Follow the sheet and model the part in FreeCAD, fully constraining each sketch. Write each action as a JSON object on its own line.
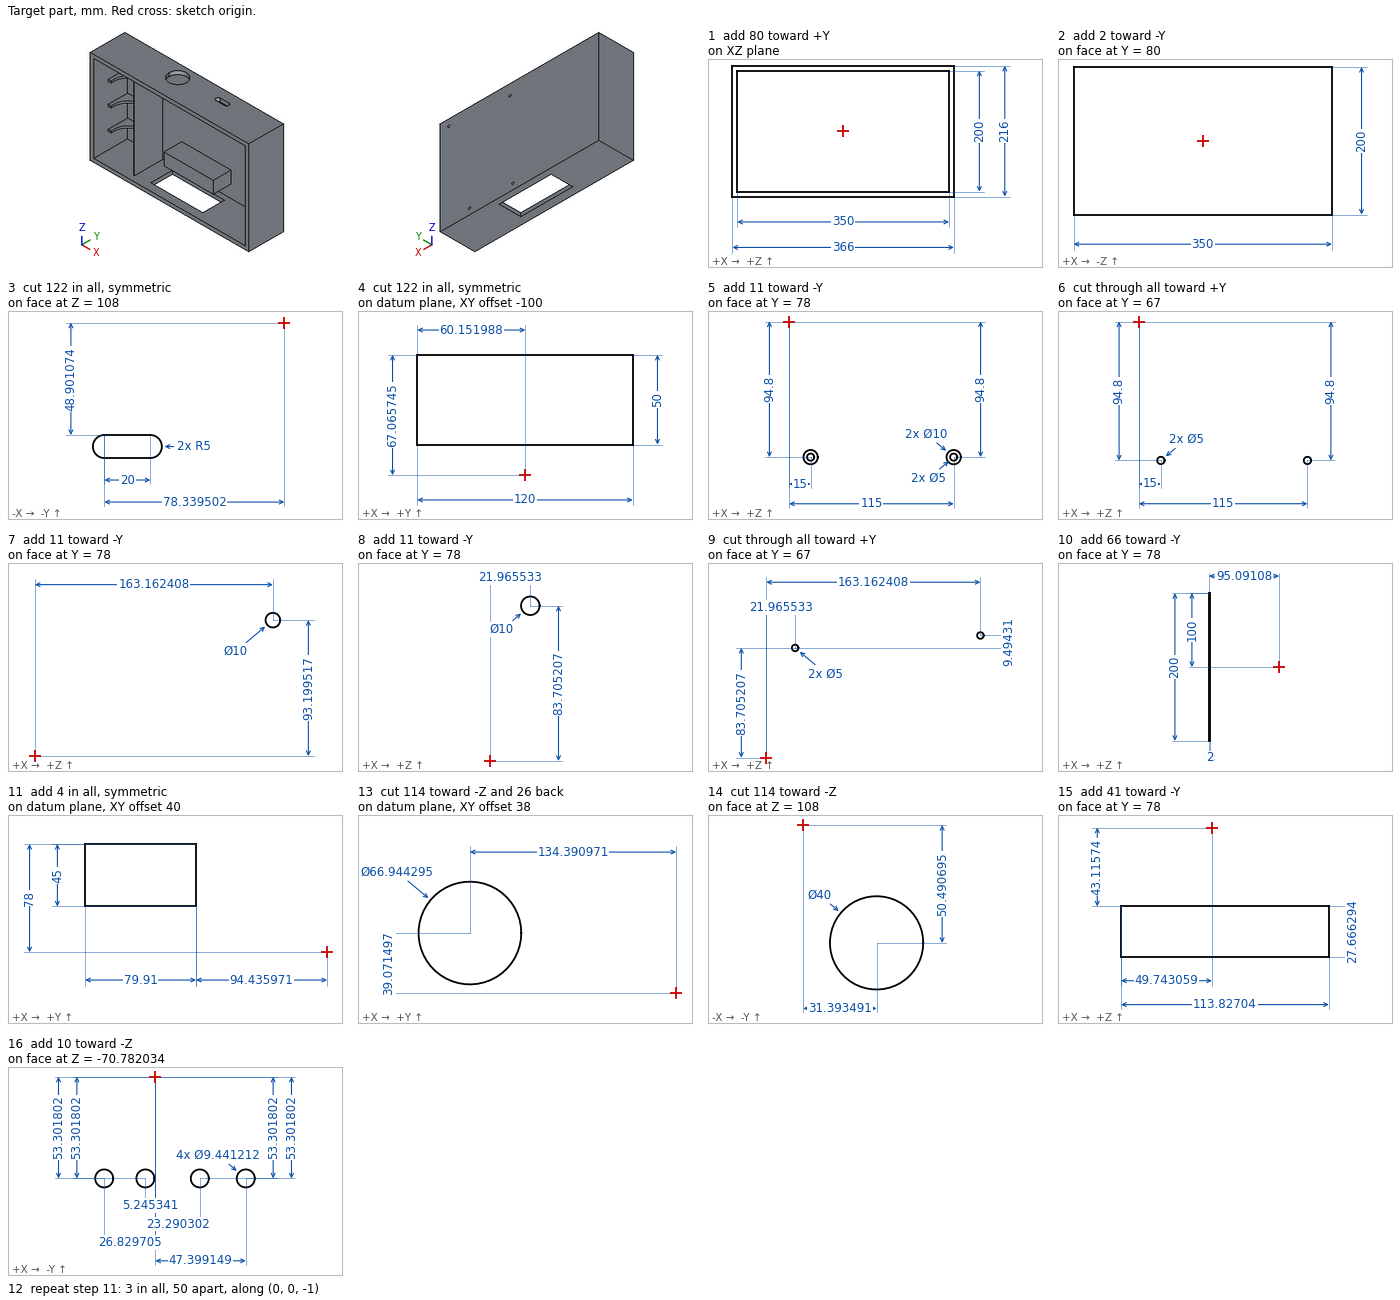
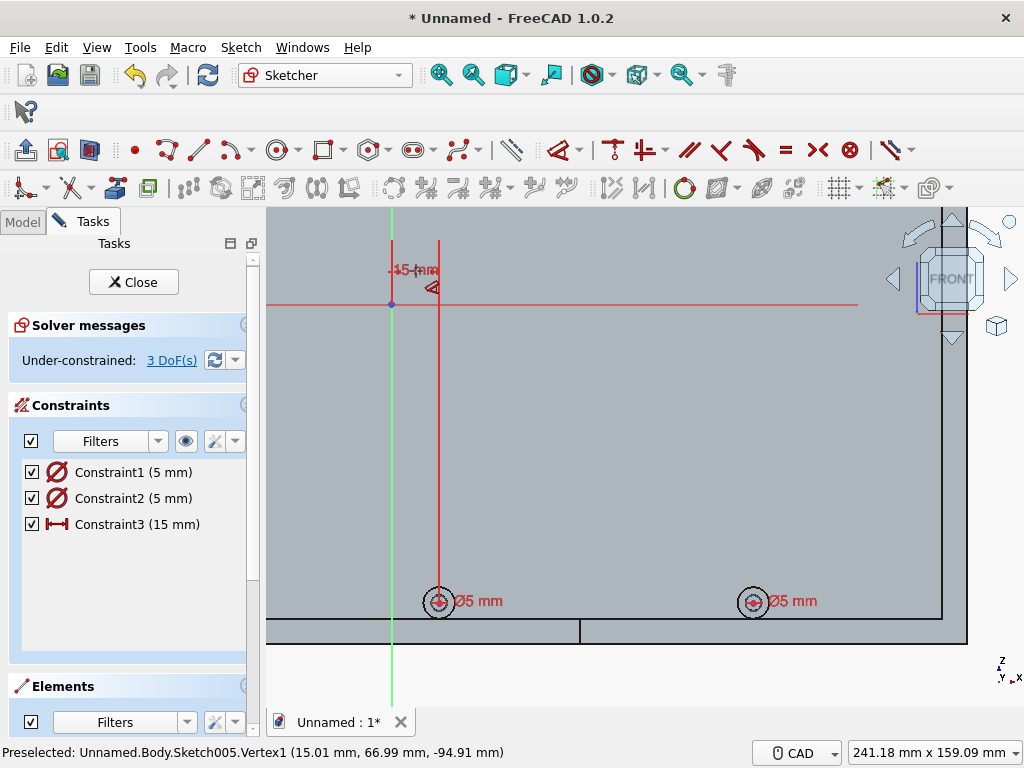
{"action": "left_click", "coordinate": [753, 603]}
{"action": "left_click", "coordinate": [573, 271]}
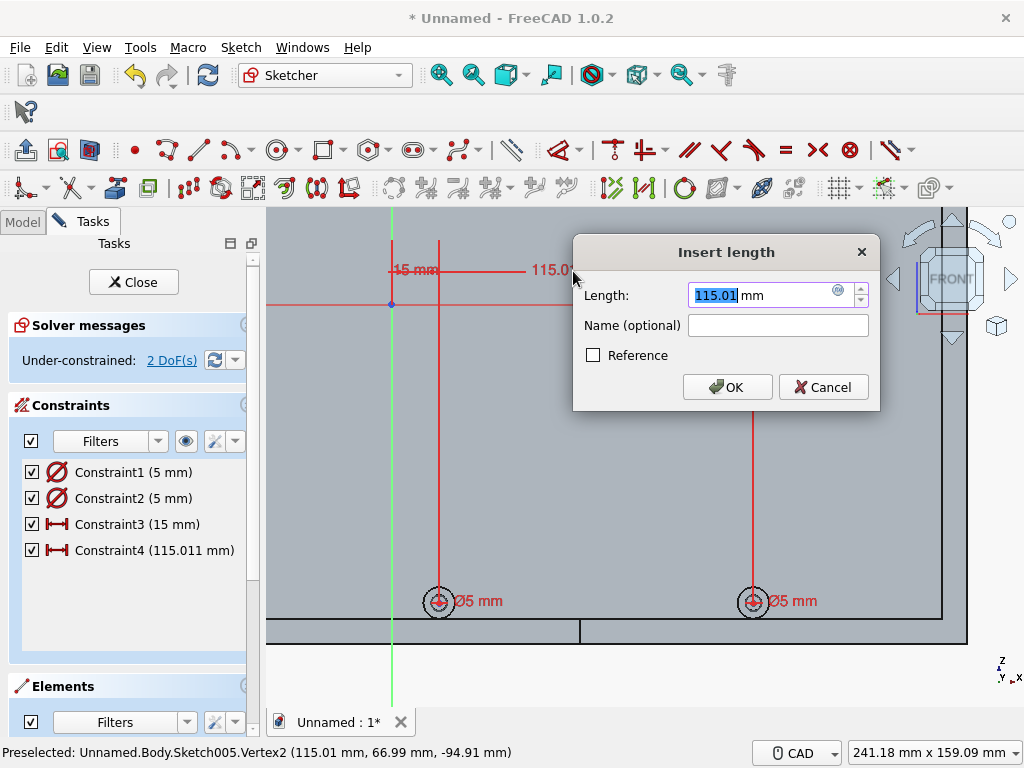
{"action": "type", "text": "115"}
{"action": "key", "text": "Return"}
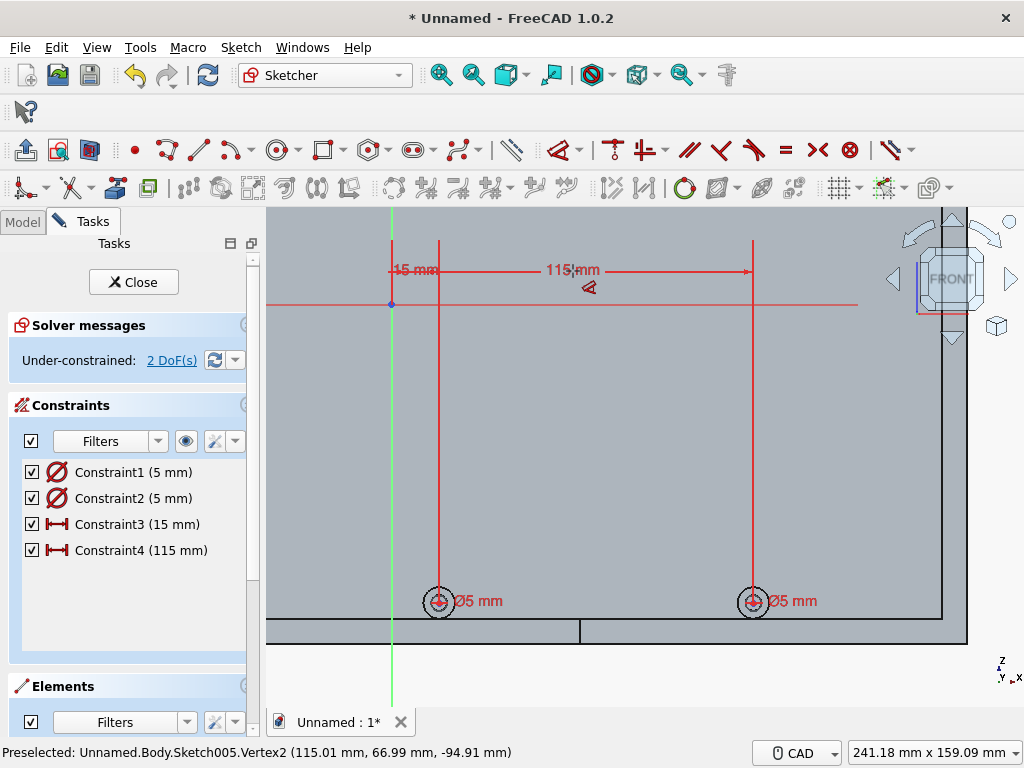
{"action": "left_click", "coordinate": [439, 603]}
{"action": "left_click", "coordinate": [358, 454]}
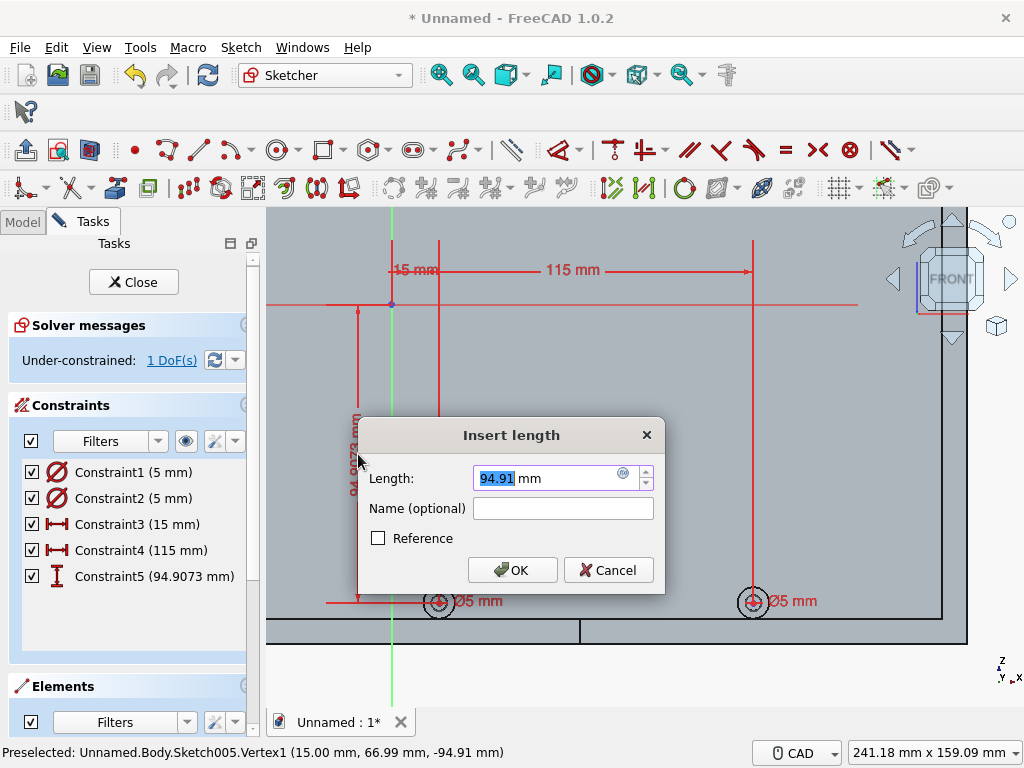
{"action": "type", "text": "94.8"}
{"action": "key", "text": "Return"}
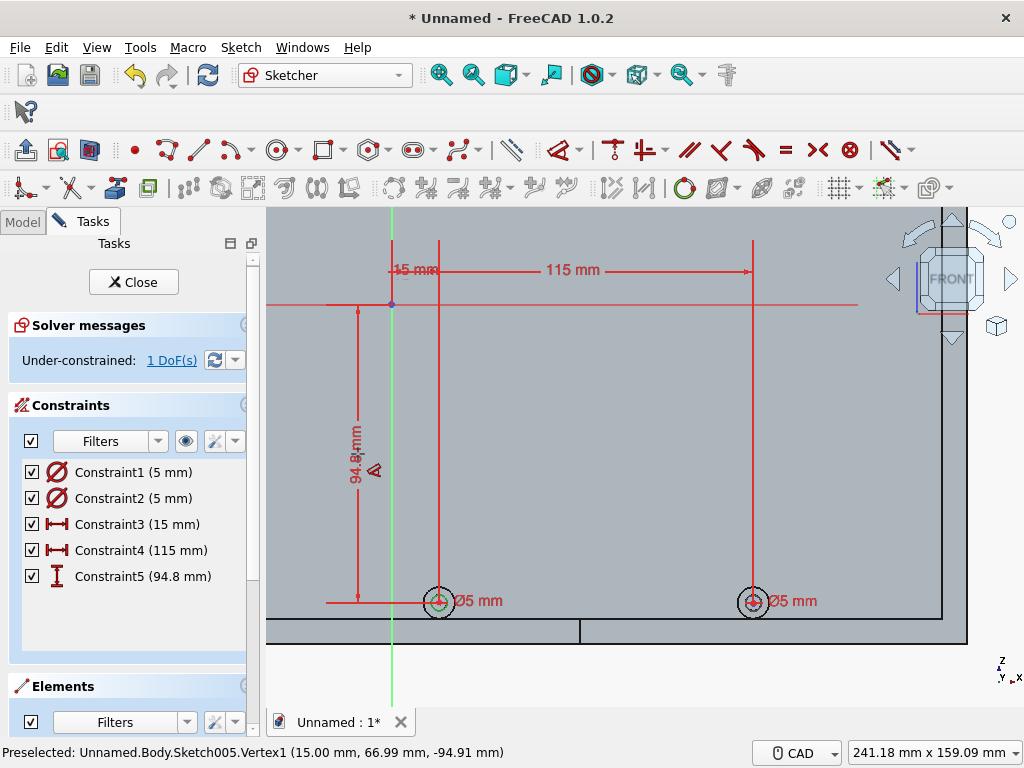
{"action": "left_click", "coordinate": [753, 603]}
{"action": "left_click", "coordinate": [358, 386]}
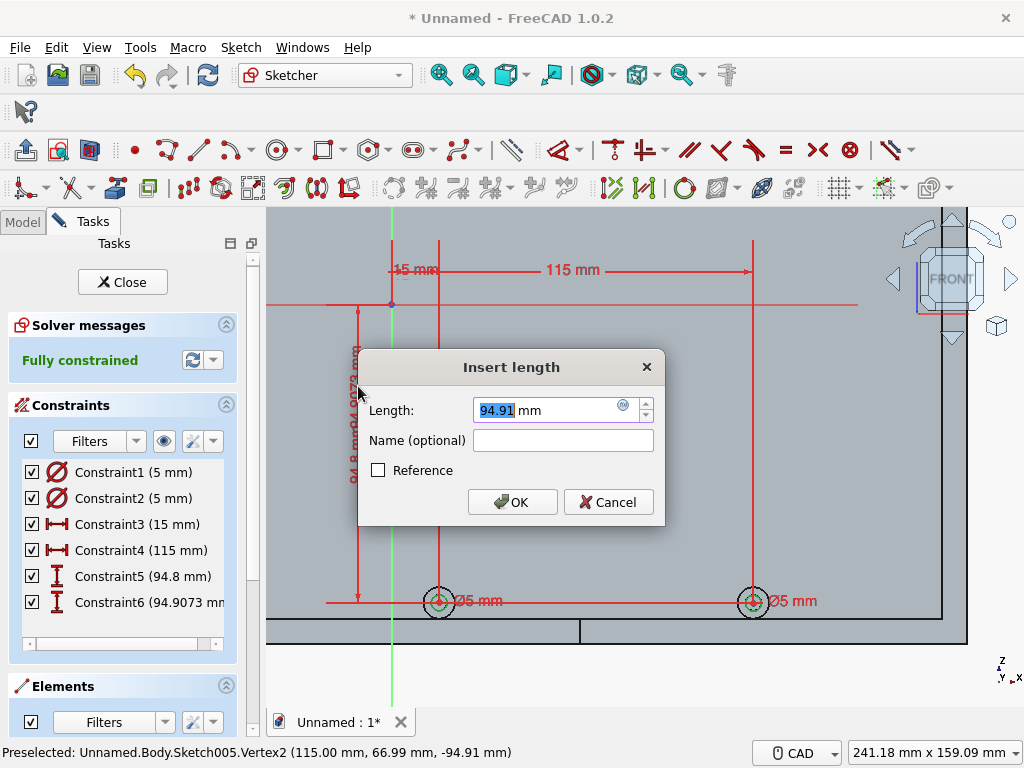
{"action": "type", "text": "94.8"}
{"action": "key", "text": "Return"}
{"action": "key", "text": "Escape"}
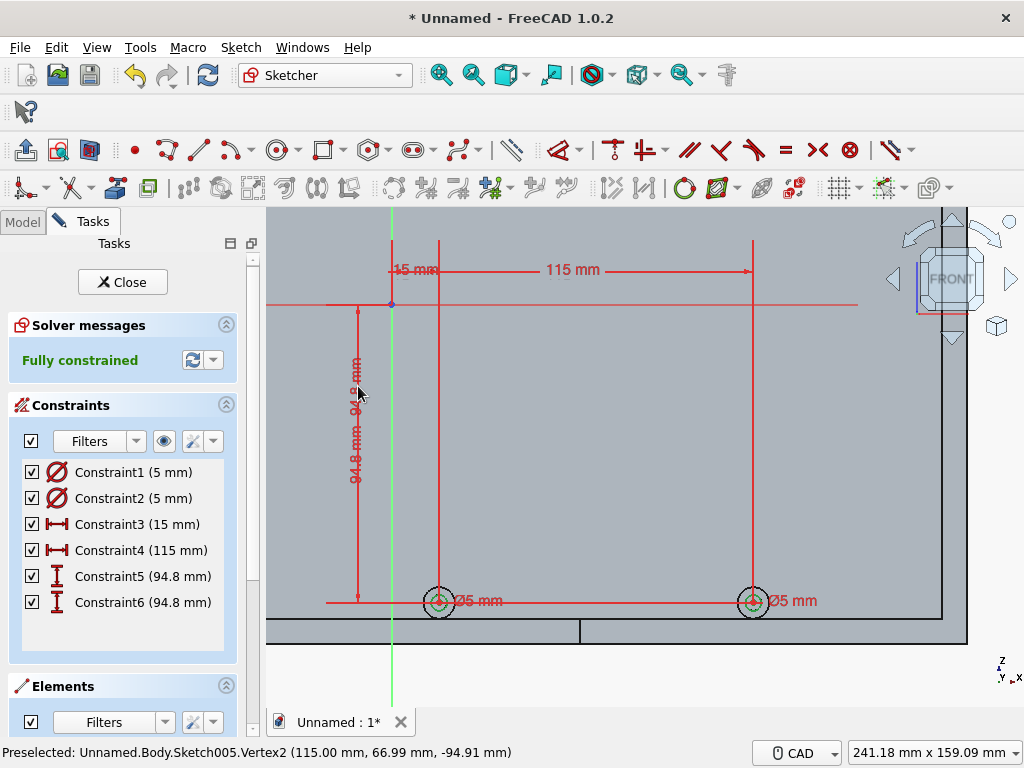
{"action": "left_click", "coordinate": [123, 282]}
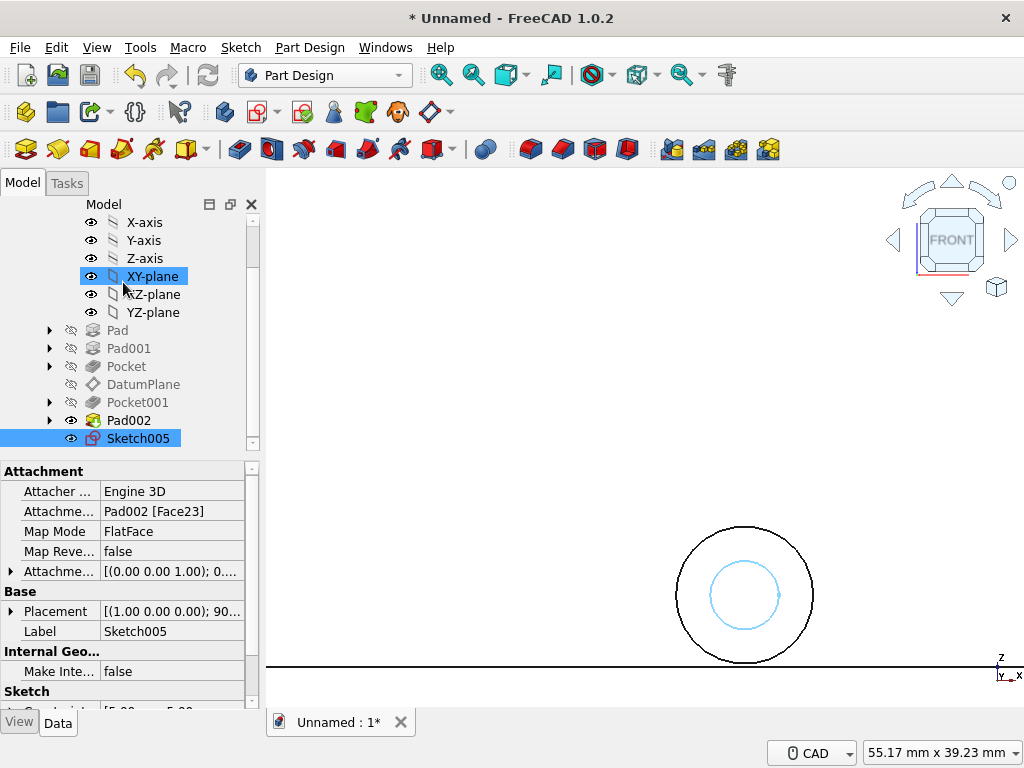
{"action": "left_click", "coordinate": [240, 150]}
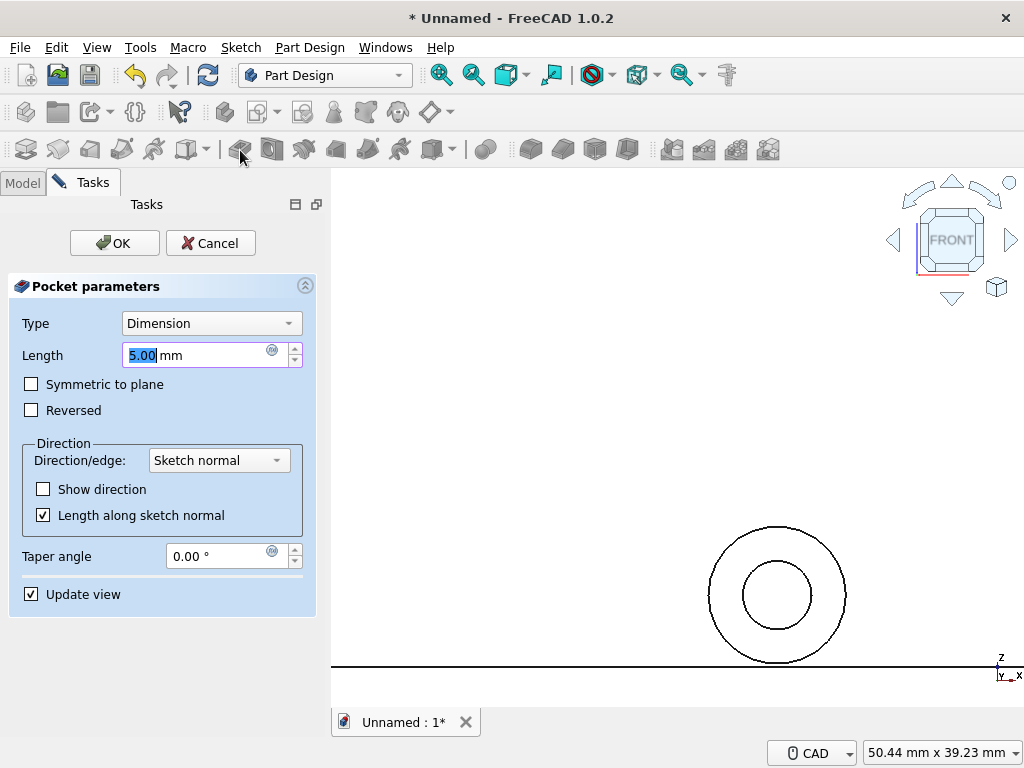
{"action": "left_click", "coordinate": [212, 324]}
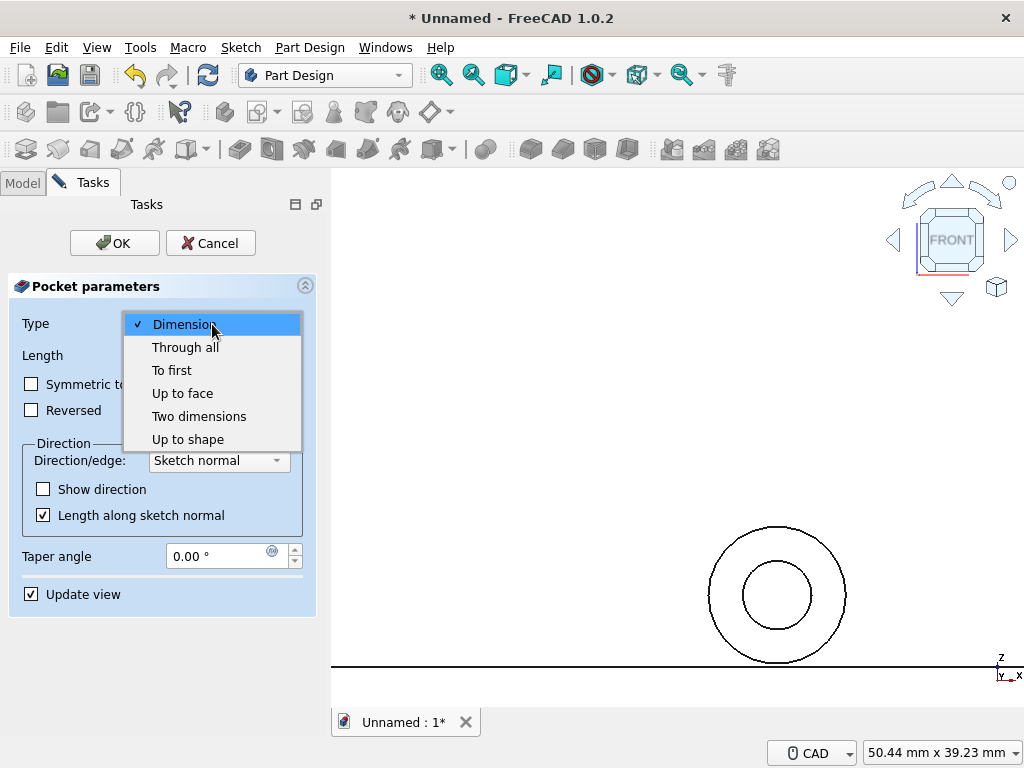
{"action": "left_click", "coordinate": [212, 348]}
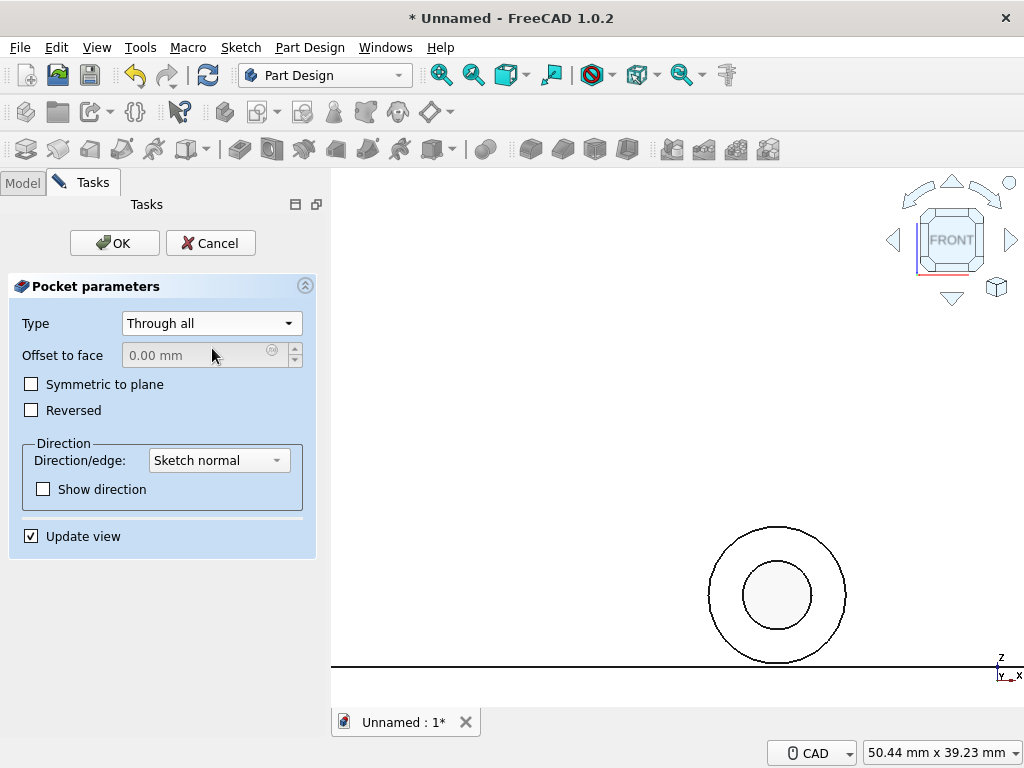
{"action": "left_click", "coordinate": [115, 243]}